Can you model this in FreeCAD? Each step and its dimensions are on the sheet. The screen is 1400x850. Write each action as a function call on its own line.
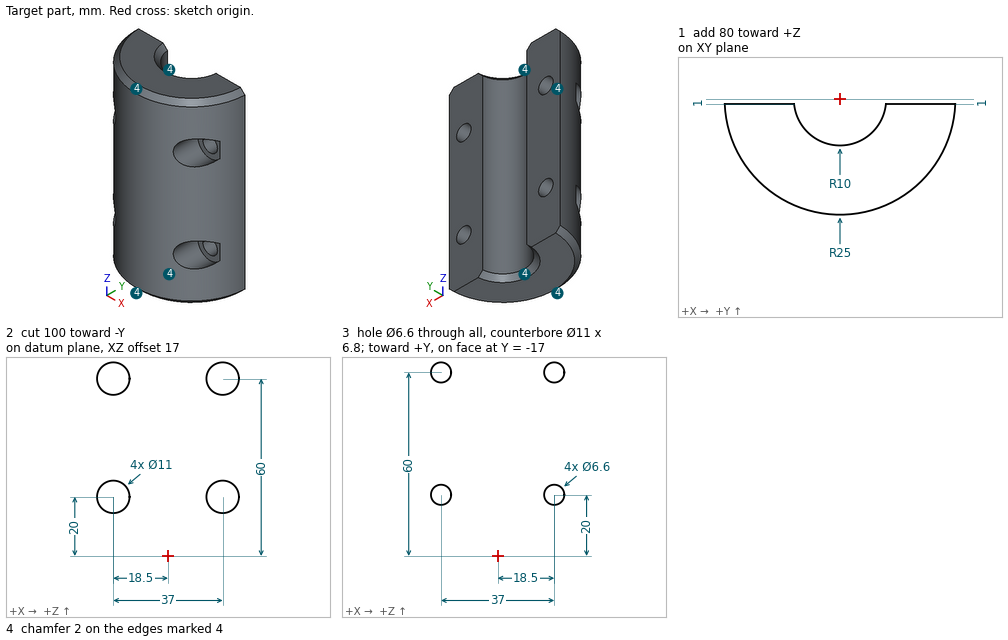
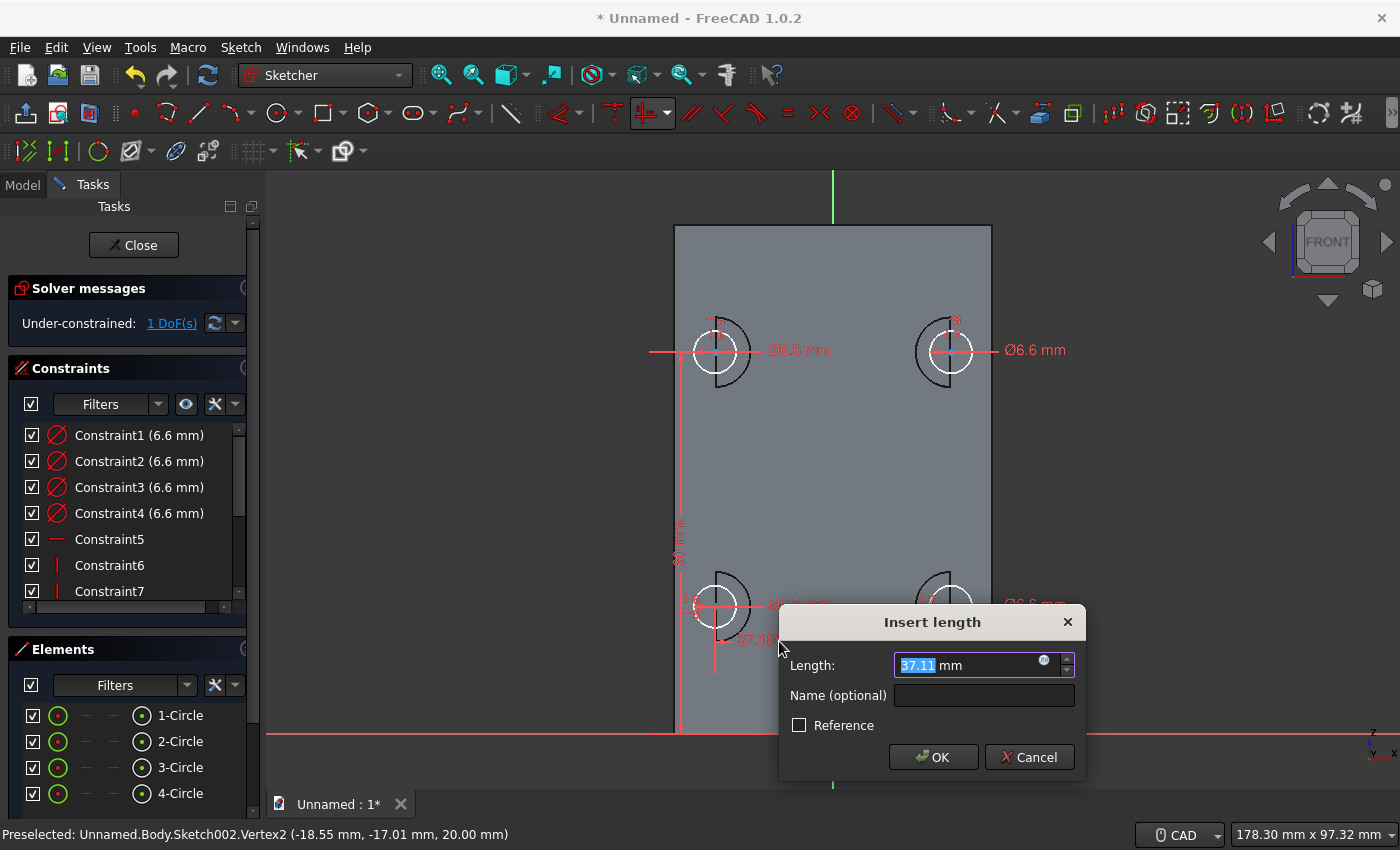
text(37)
key(Return)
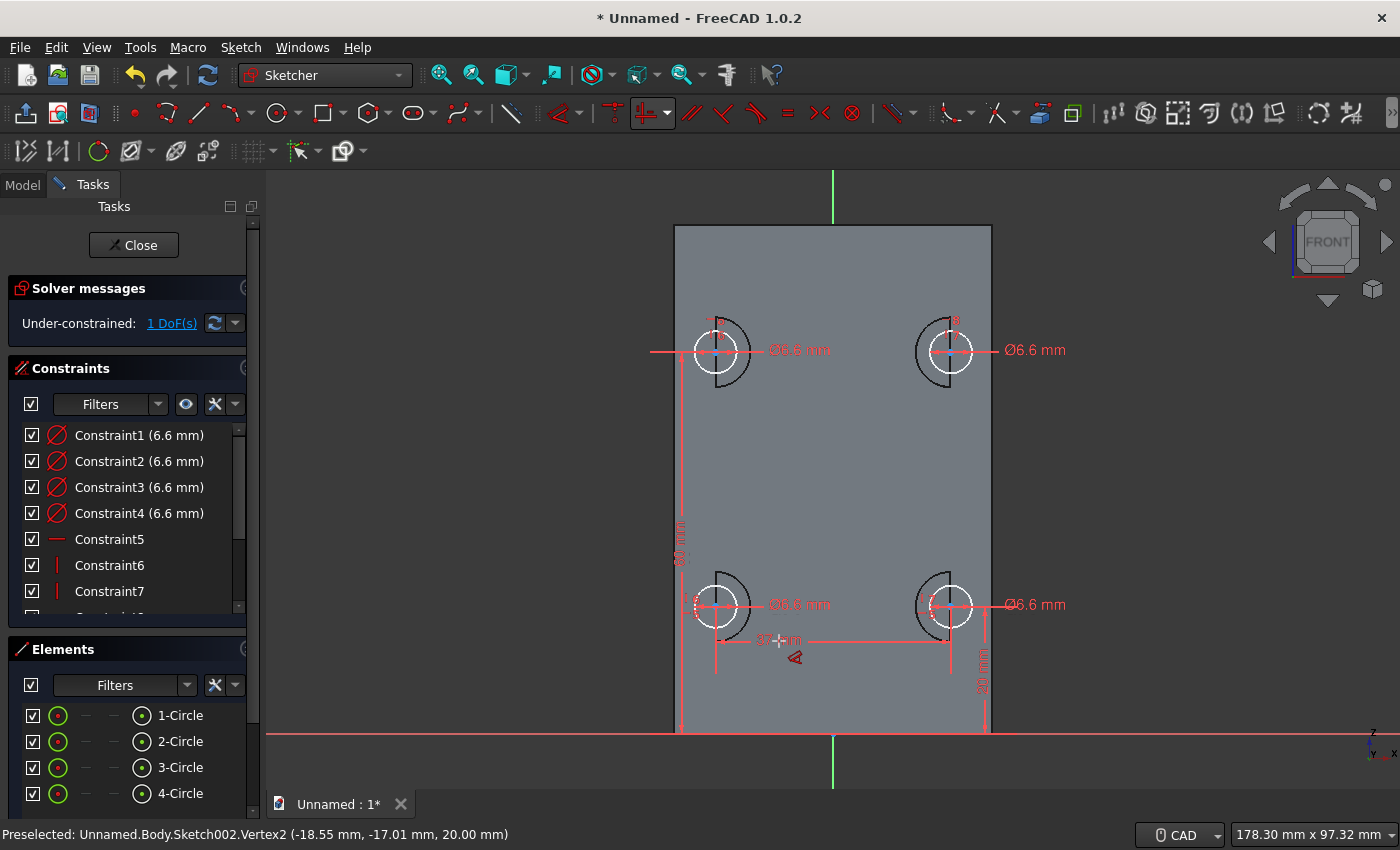
click(951, 607)
click(892, 573)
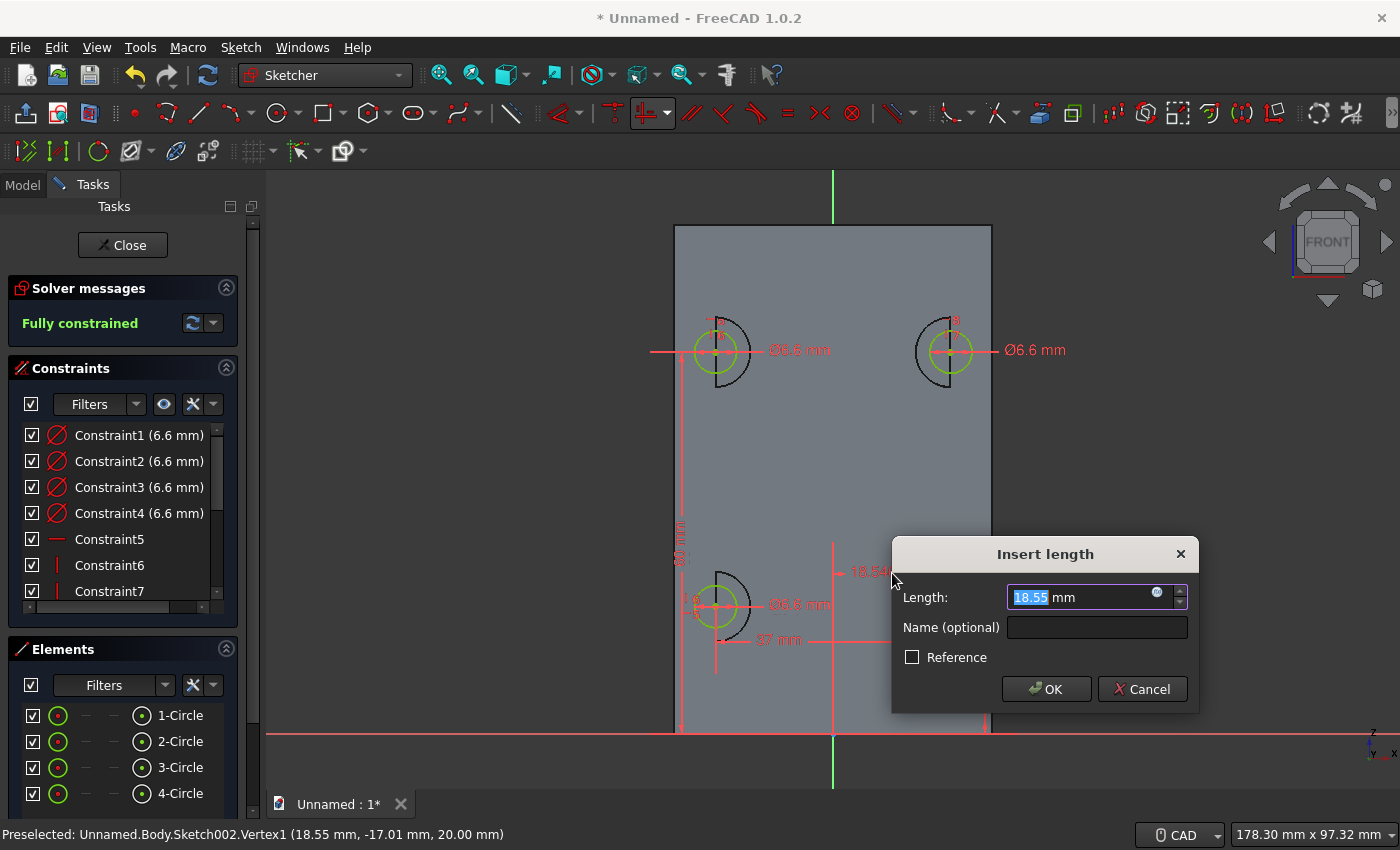
text(18.5)
key(Return)
key(Escape)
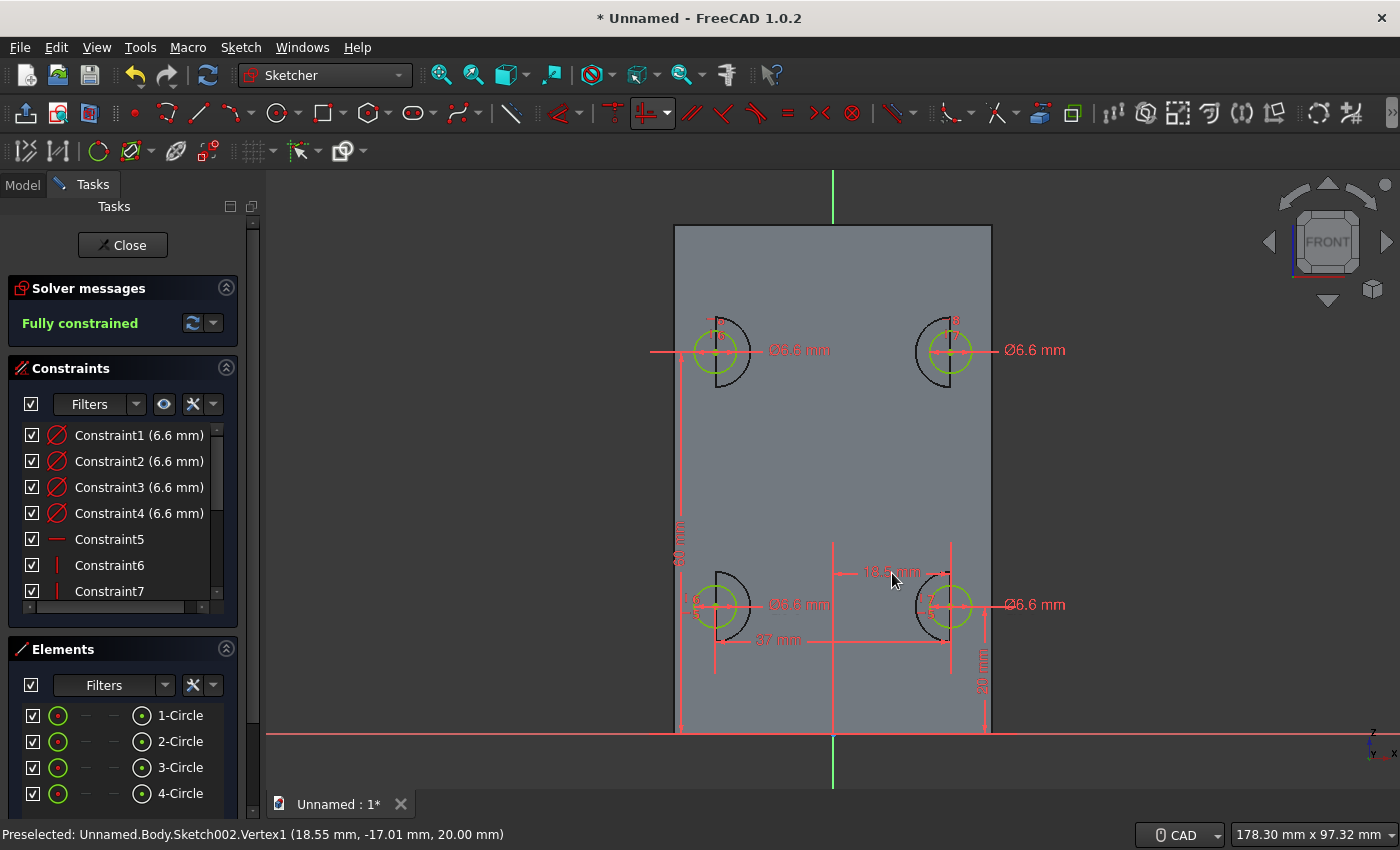
click(123, 245)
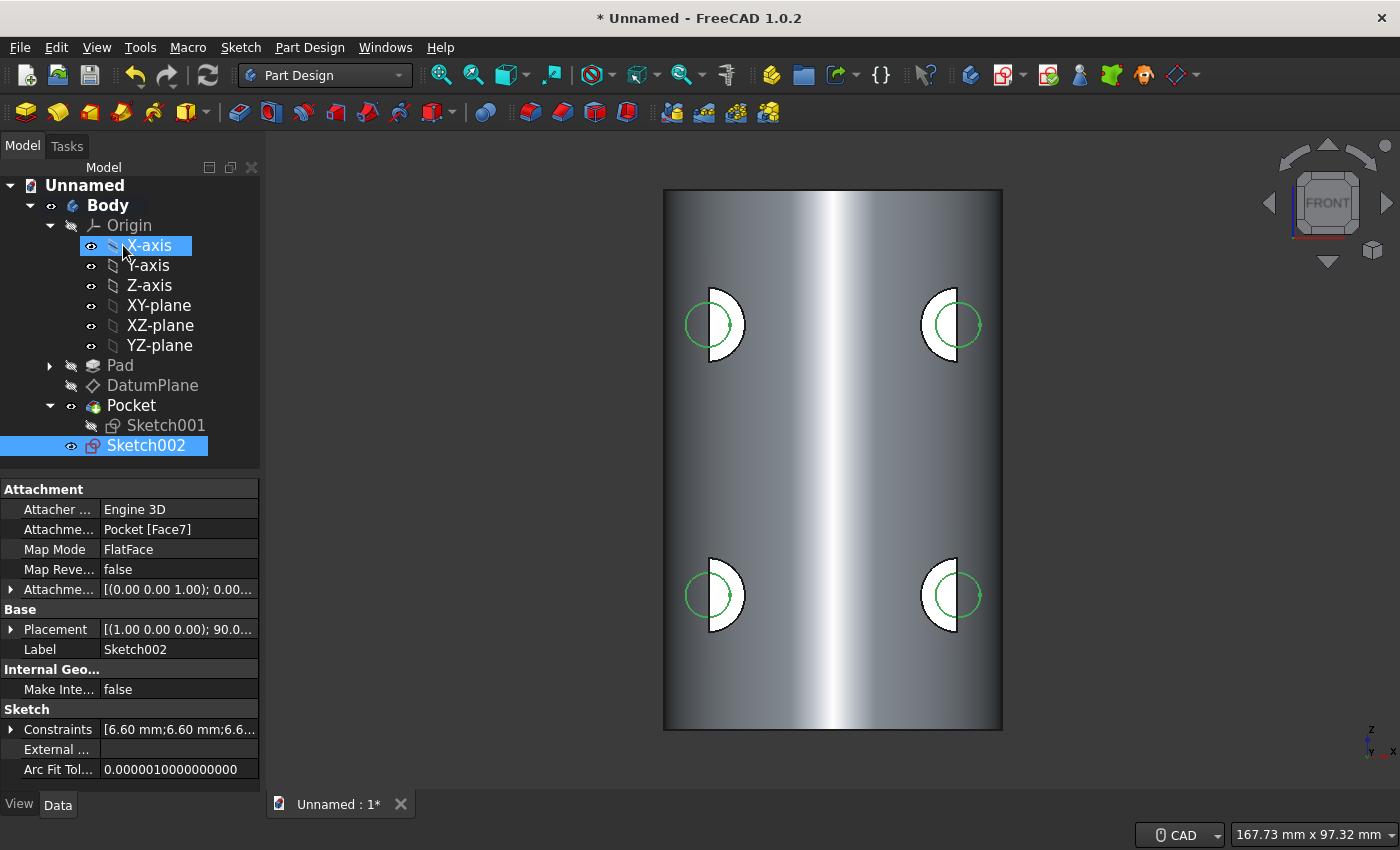
click(272, 112)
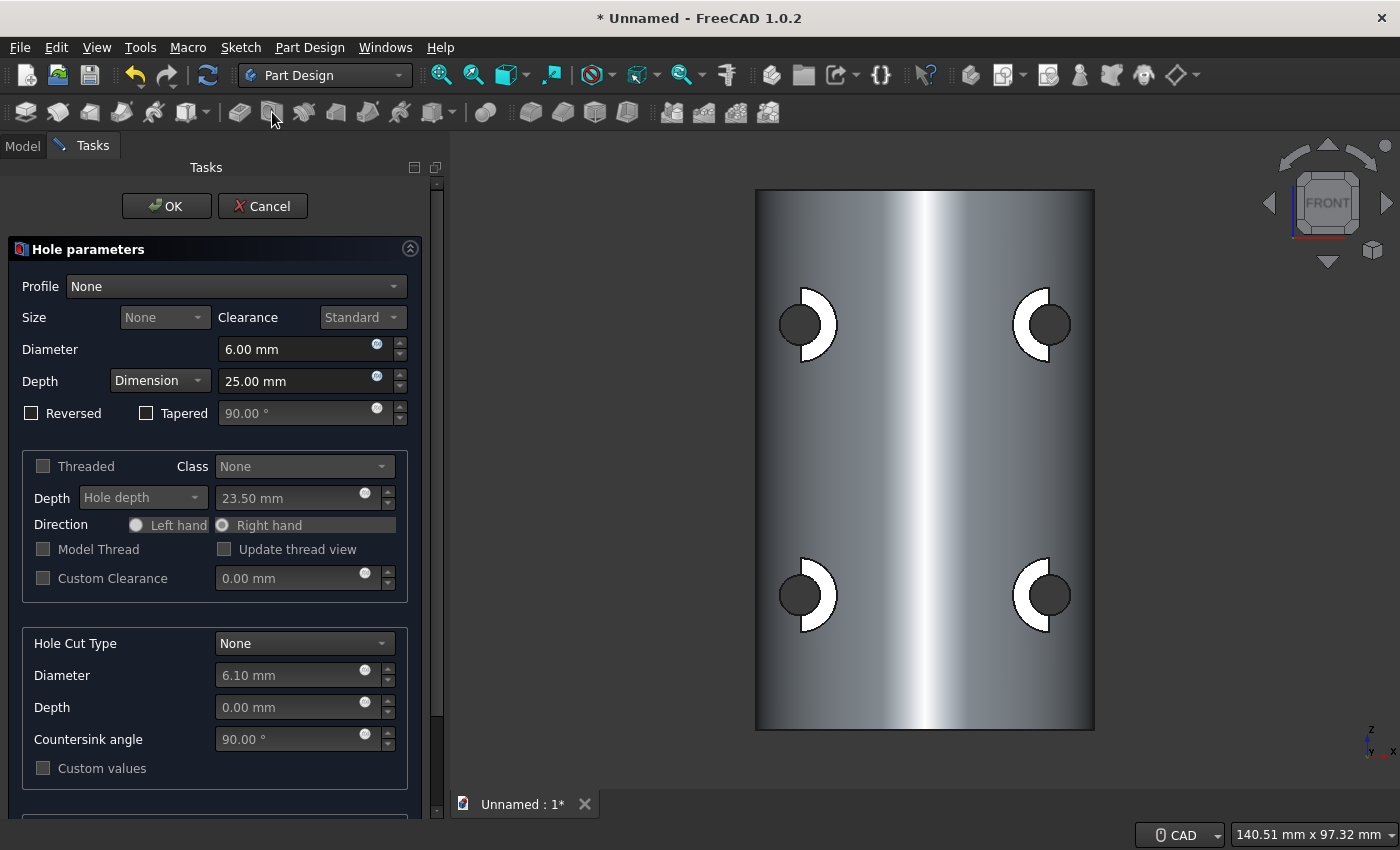
triple_click(305, 349)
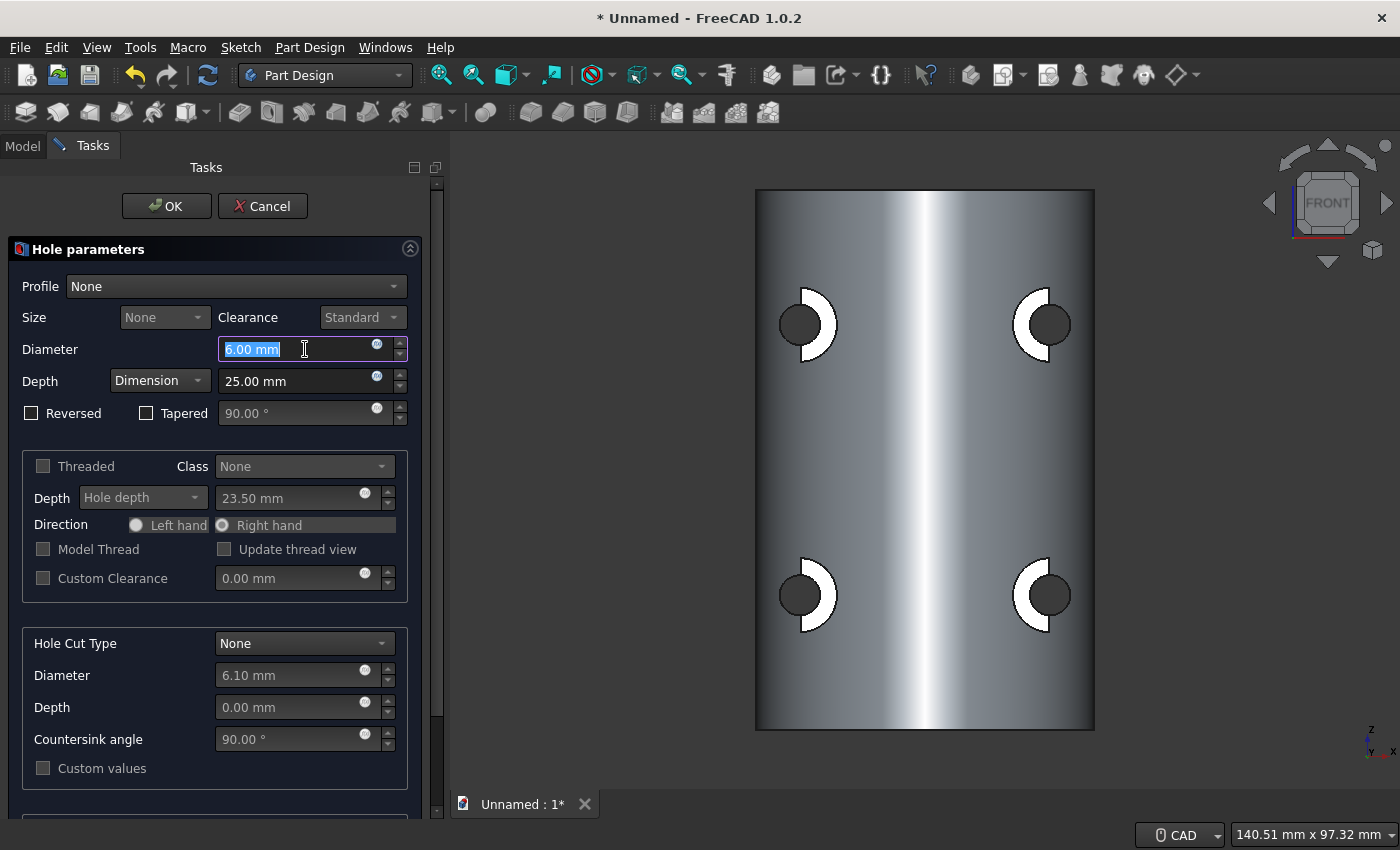
text(6.6)
key(Tab)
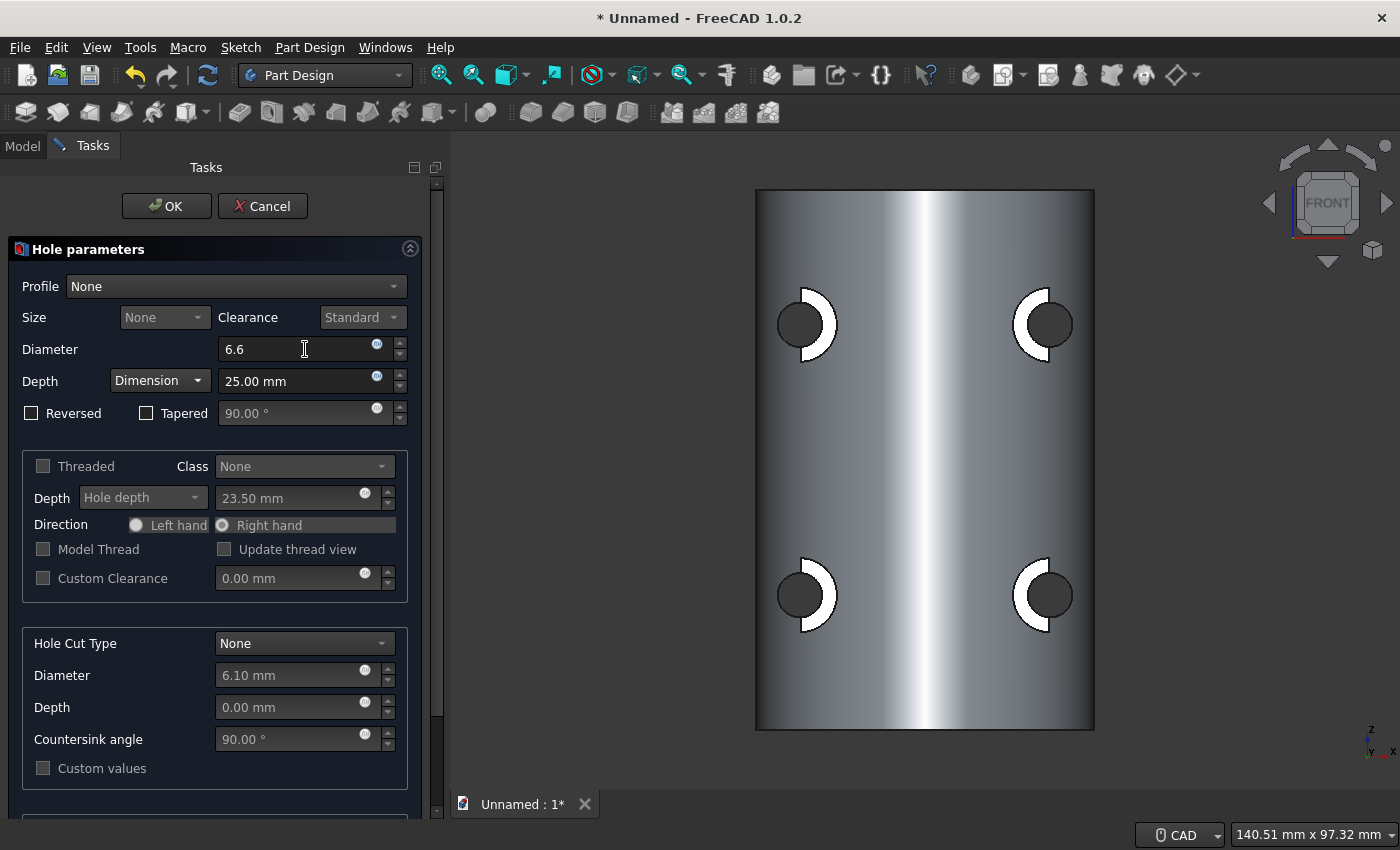
click(161, 380)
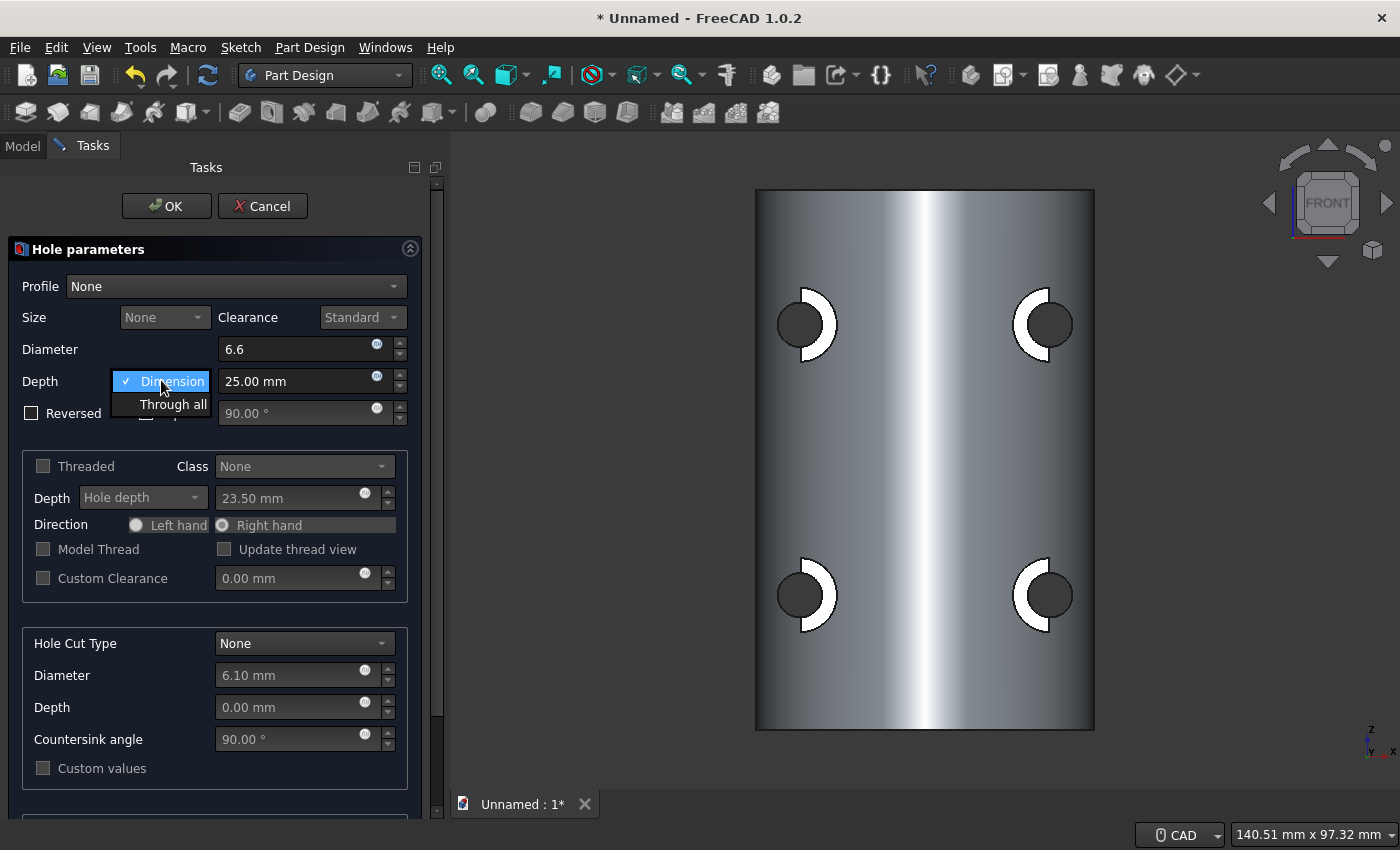
click(160, 404)